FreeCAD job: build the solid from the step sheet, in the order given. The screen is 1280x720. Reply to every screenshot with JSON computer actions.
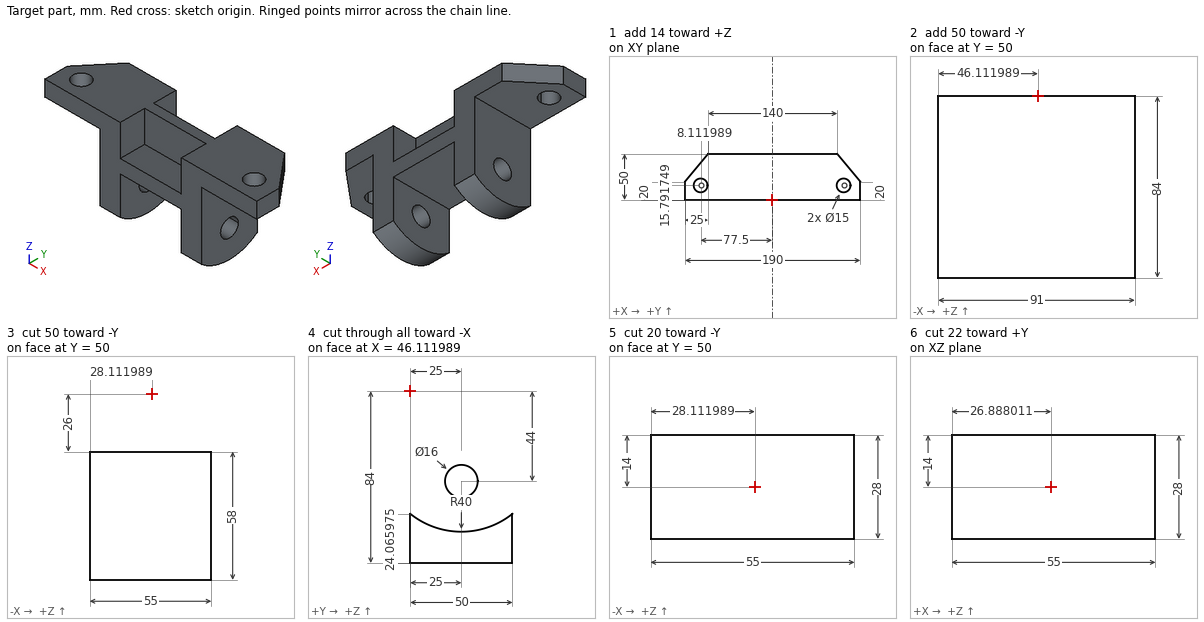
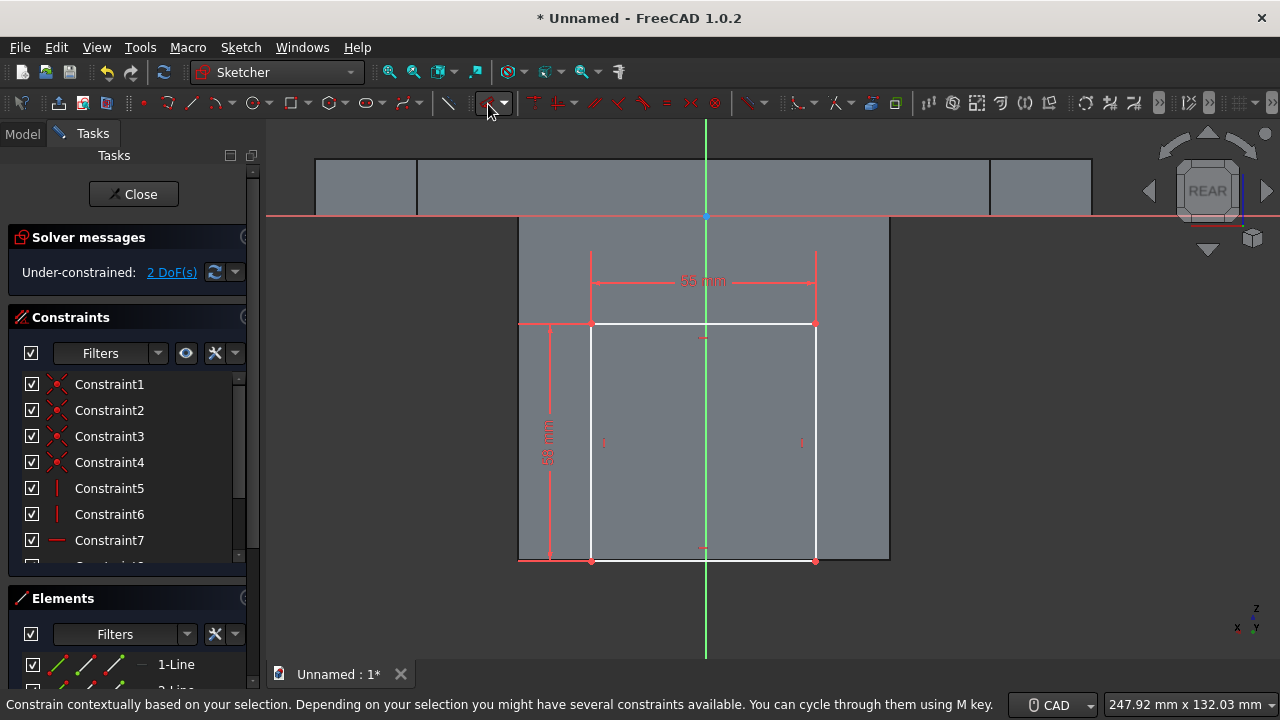
{"action": "left_click", "coordinate": [591, 324]}
{"action": "left_click", "coordinate": [557, 270]}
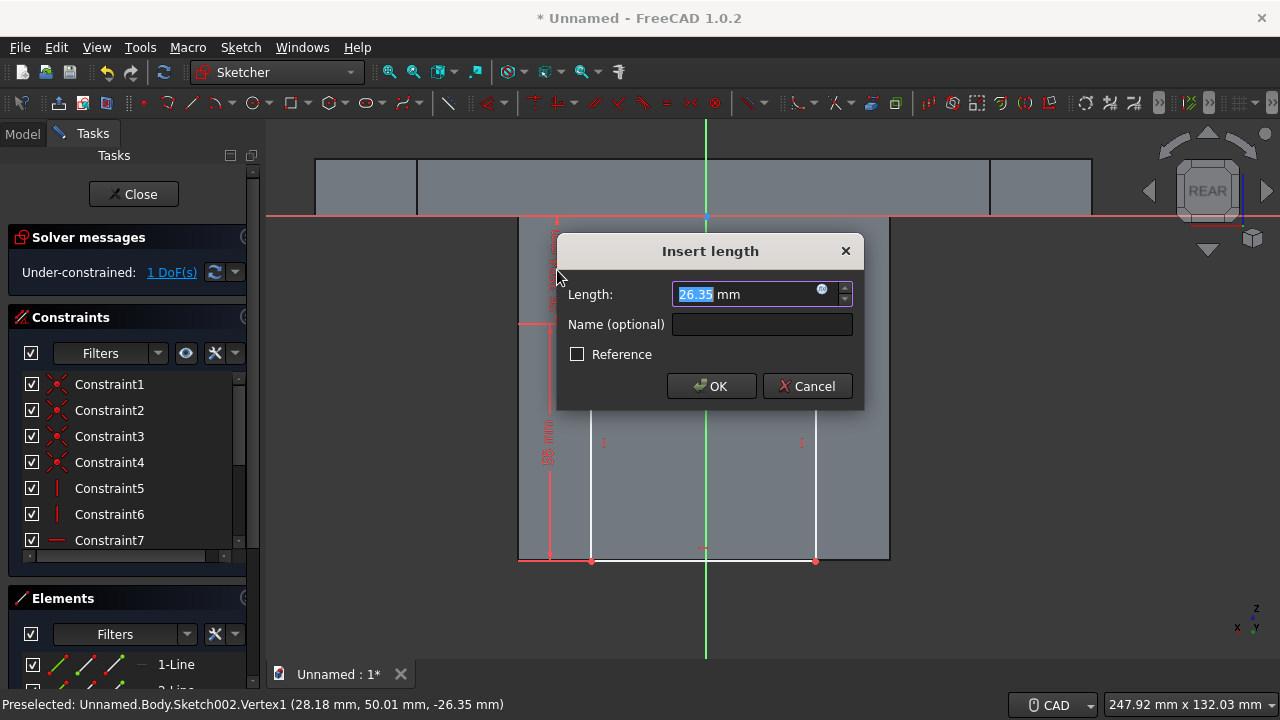
{"action": "type", "text": "26"}
{"action": "key", "text": "Return"}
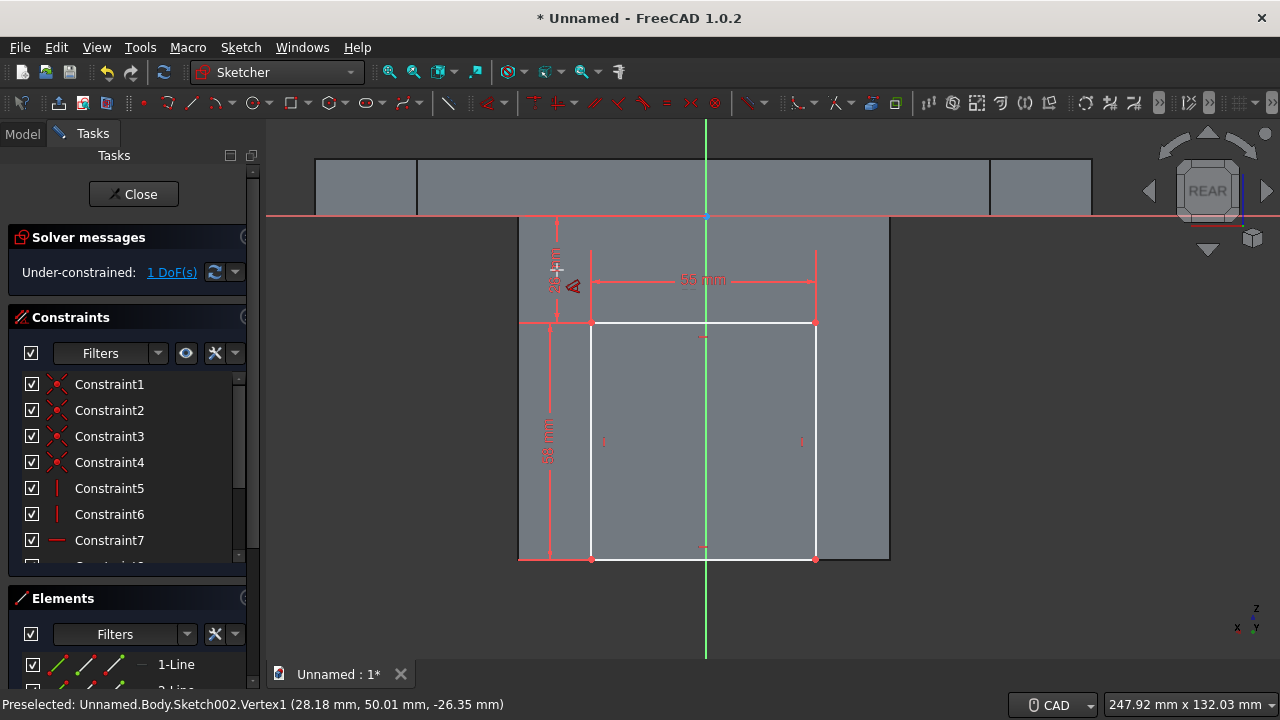
{"action": "left_click", "coordinate": [591, 323]}
{"action": "left_click", "coordinate": [649, 182]}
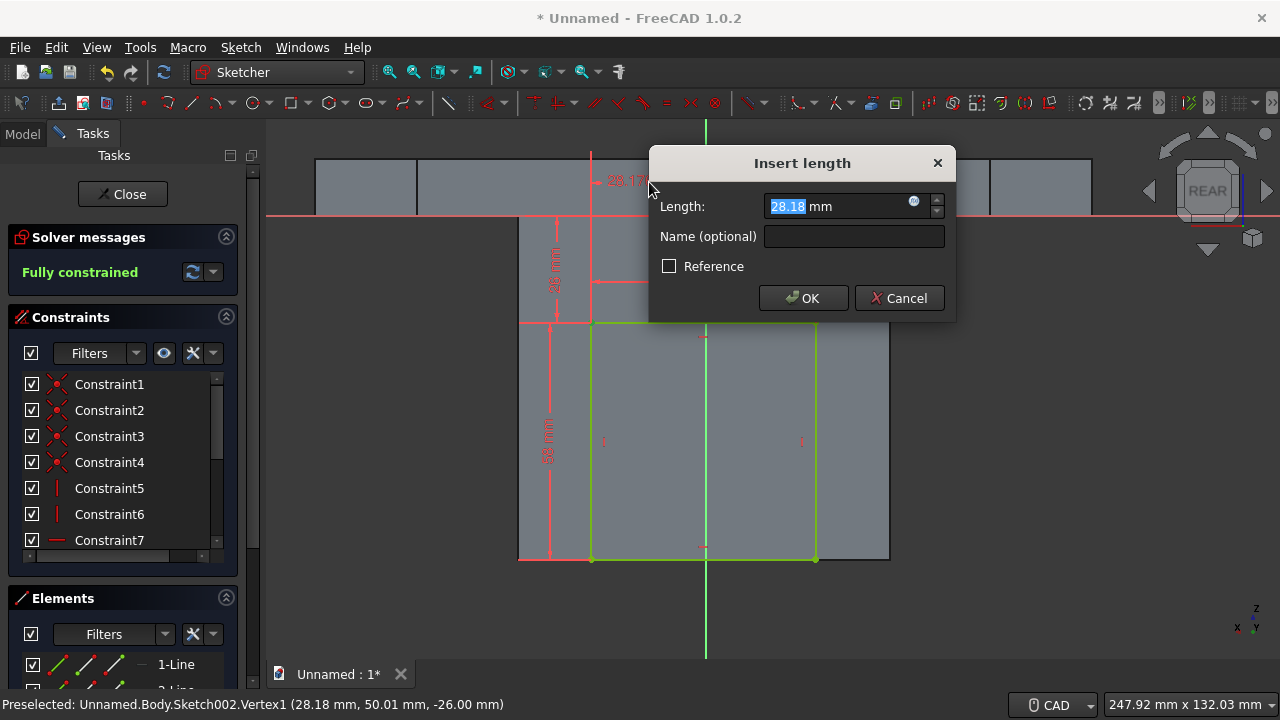
{"action": "type", "text": "28.111989"}
{"action": "key", "text": "Return"}
{"action": "key", "text": "Escape"}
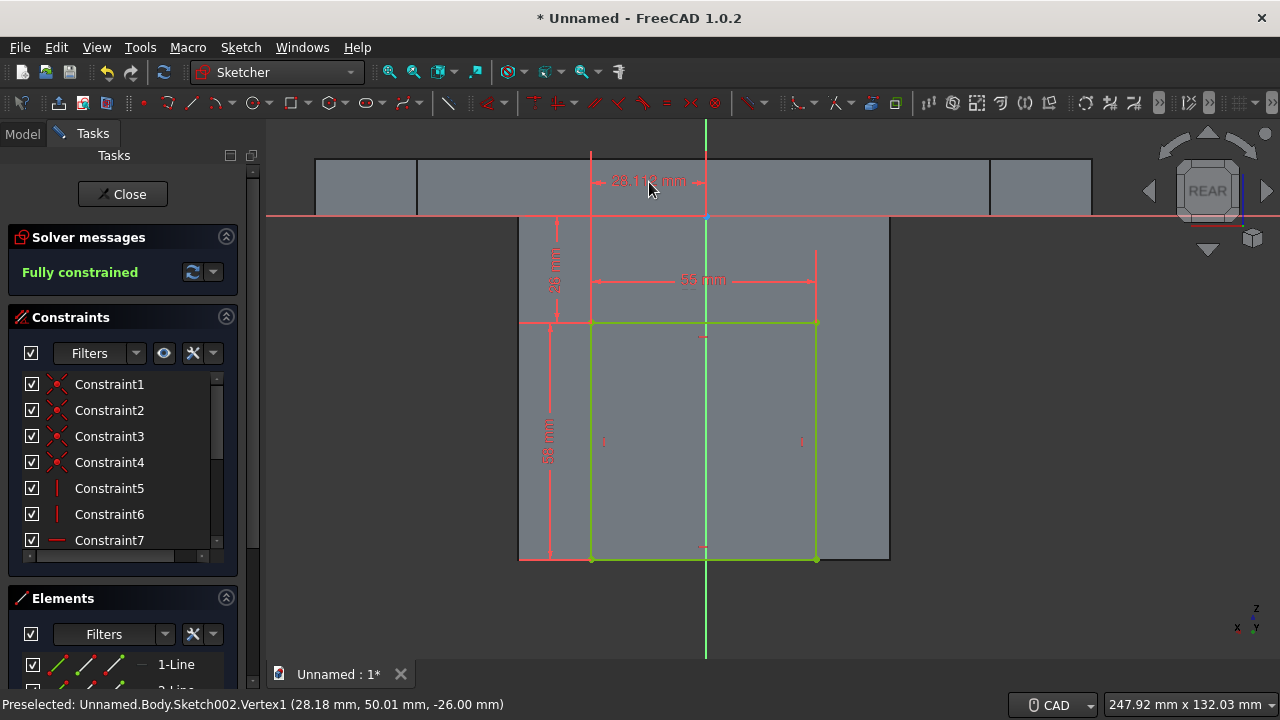
{"action": "left_click", "coordinate": [123, 194]}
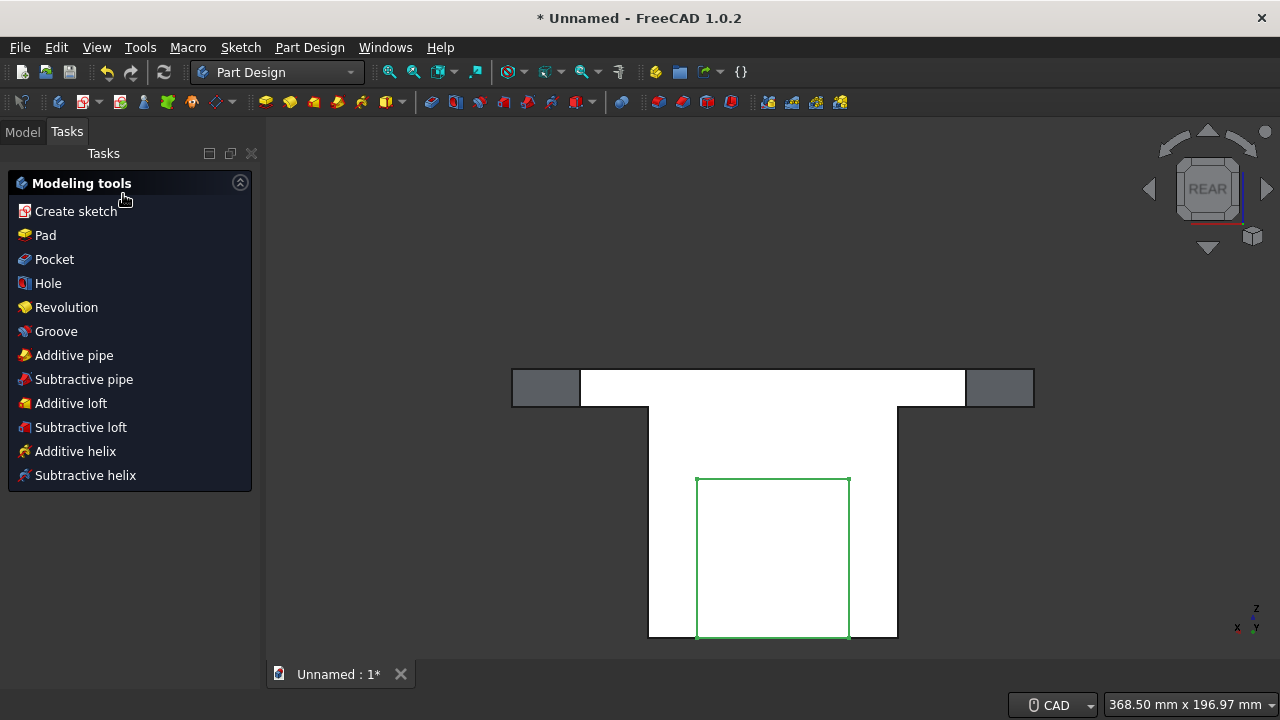
{"action": "left_click", "coordinate": [432, 102]}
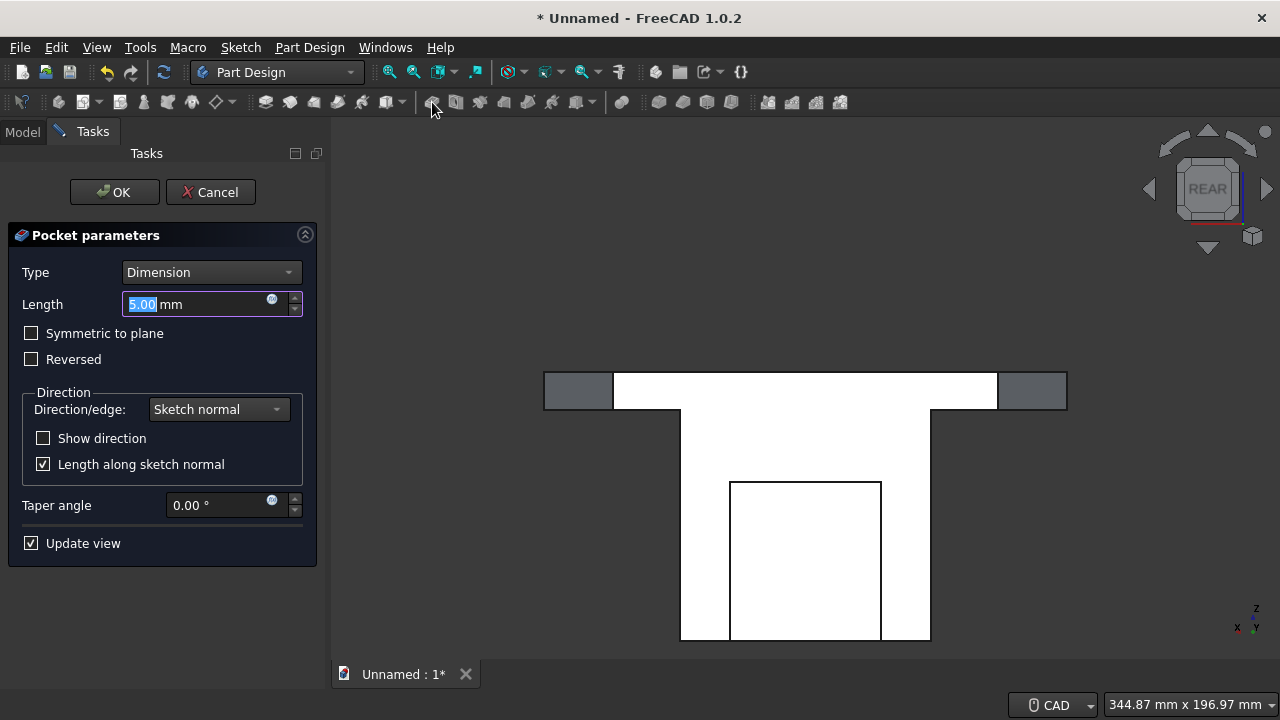
{"action": "type", "text": "50"}
{"action": "key", "text": "Tab"}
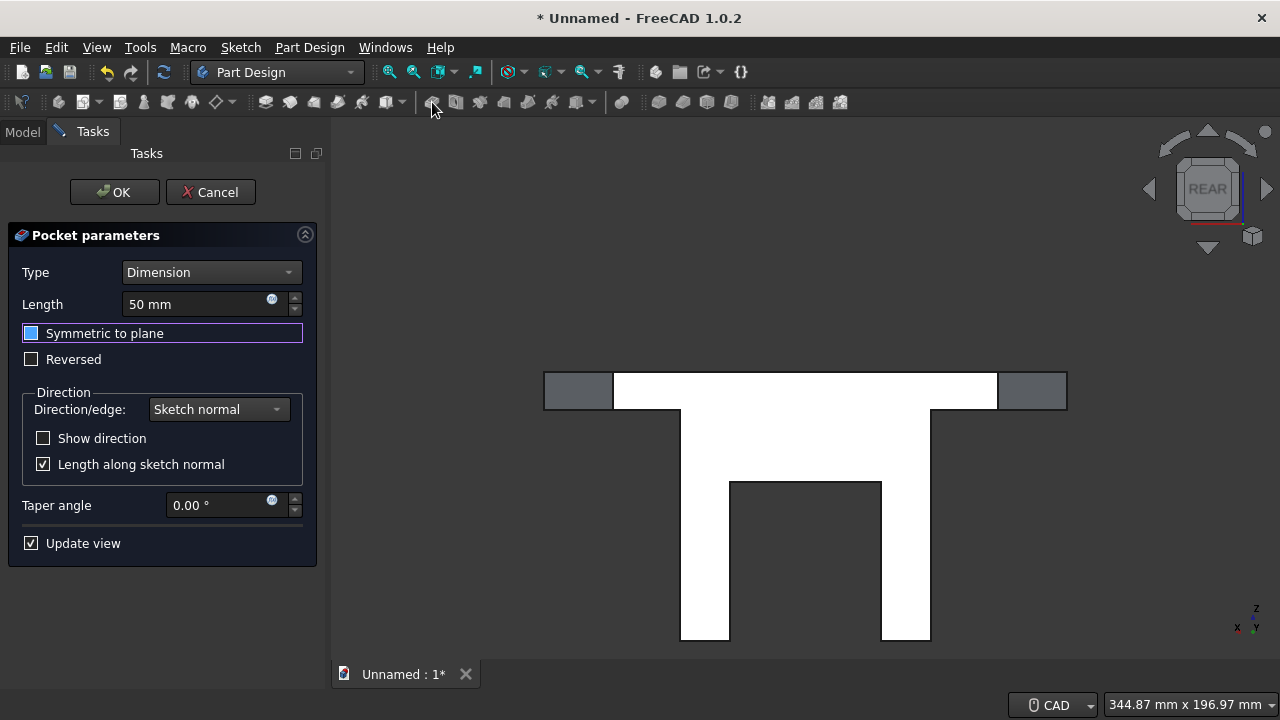
{"action": "left_click", "coordinate": [115, 192]}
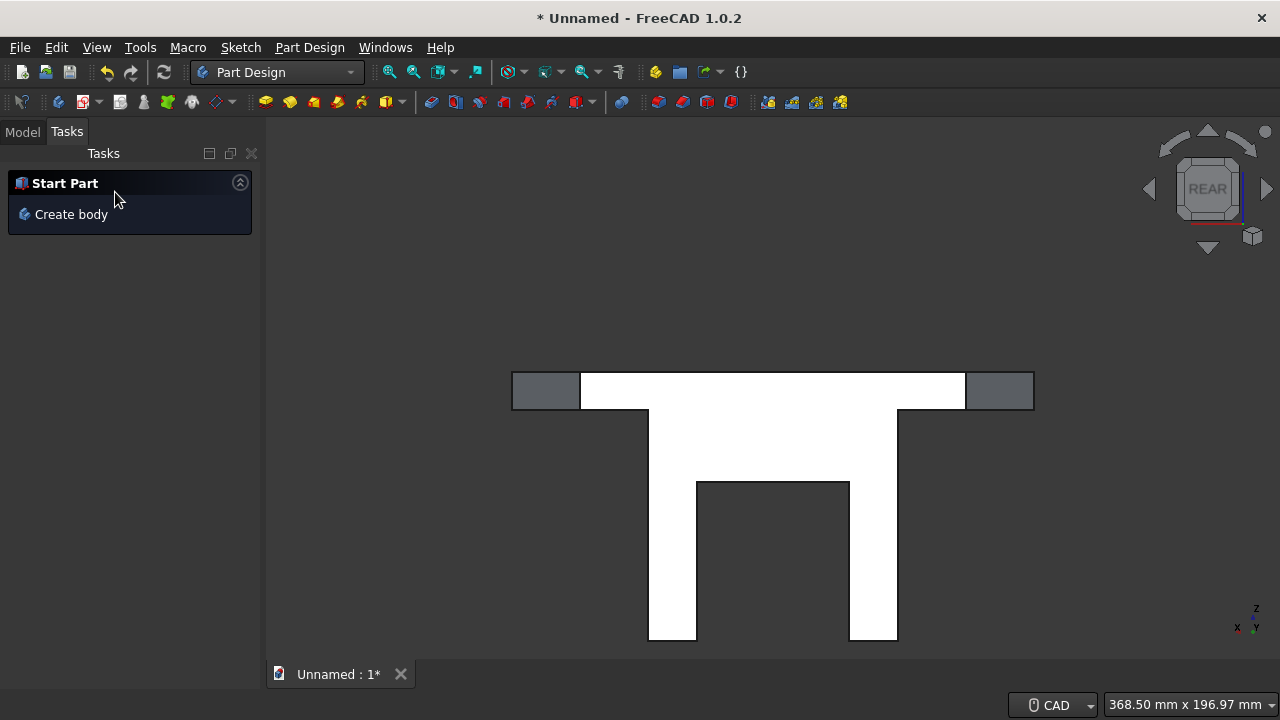
{"action": "key", "text": "0"}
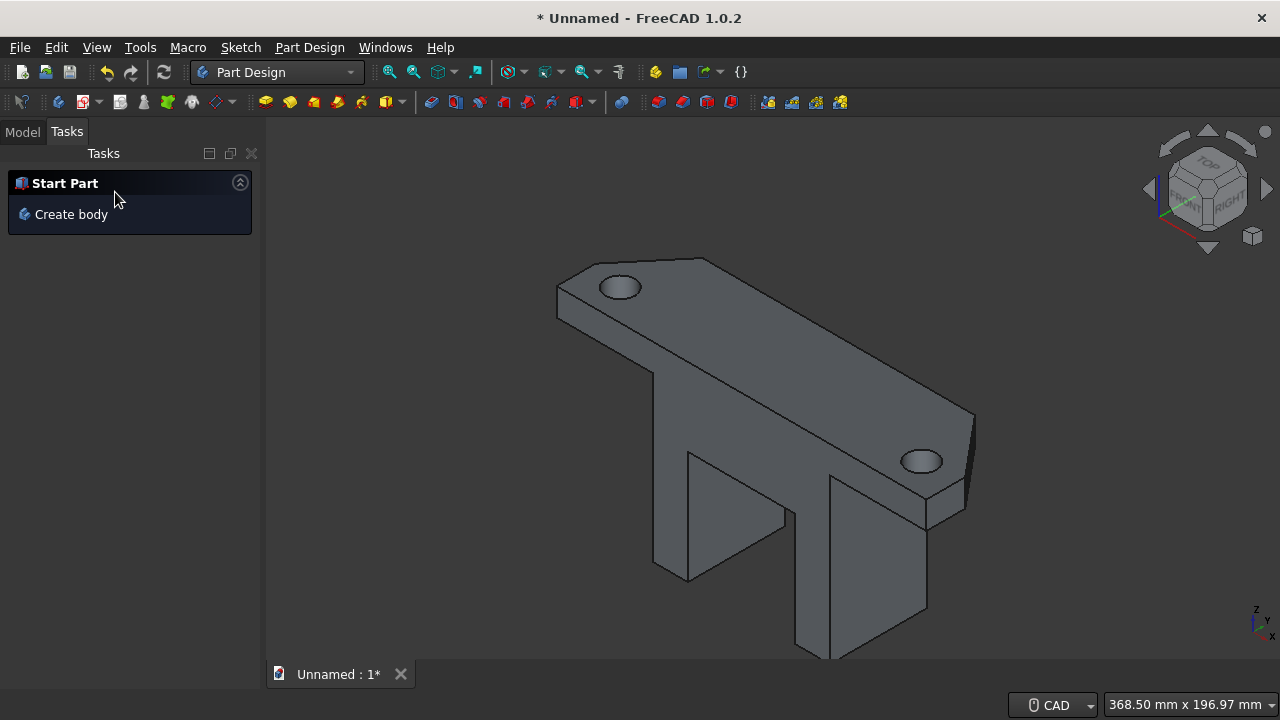
{"action": "left_click", "coordinate": [390, 72]}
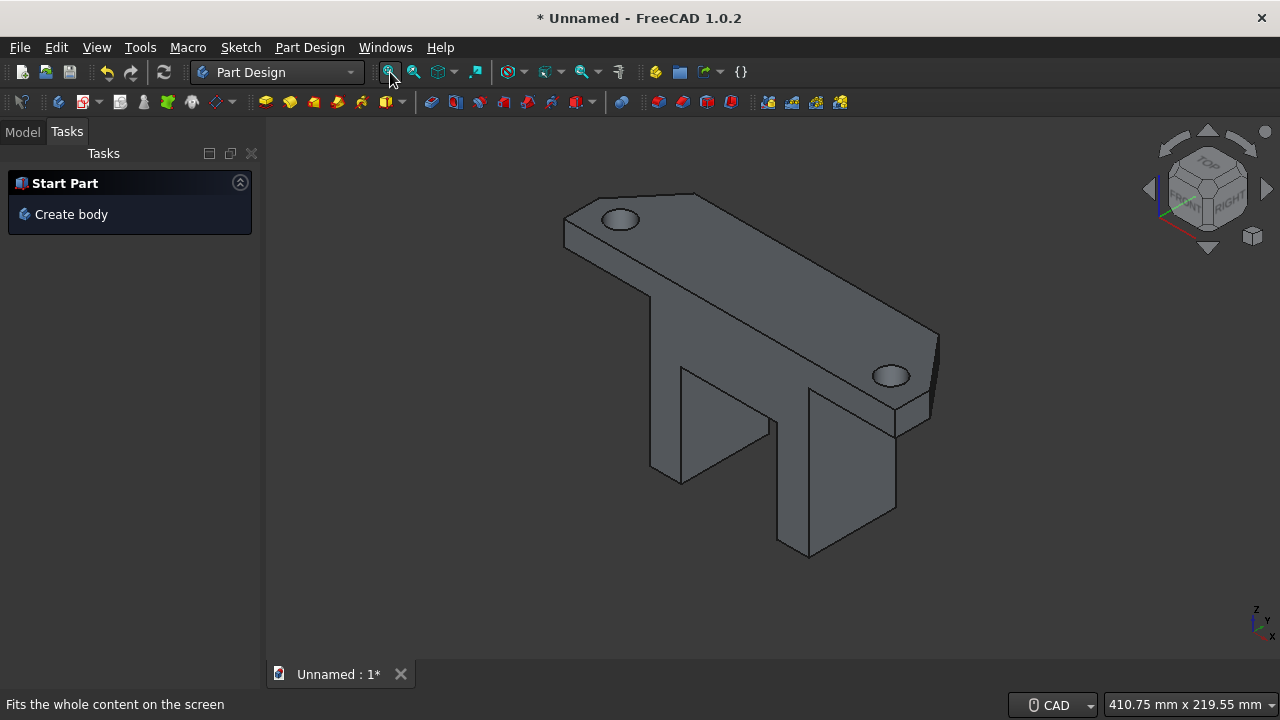
{"action": "left_click", "coordinate": [852, 423]}